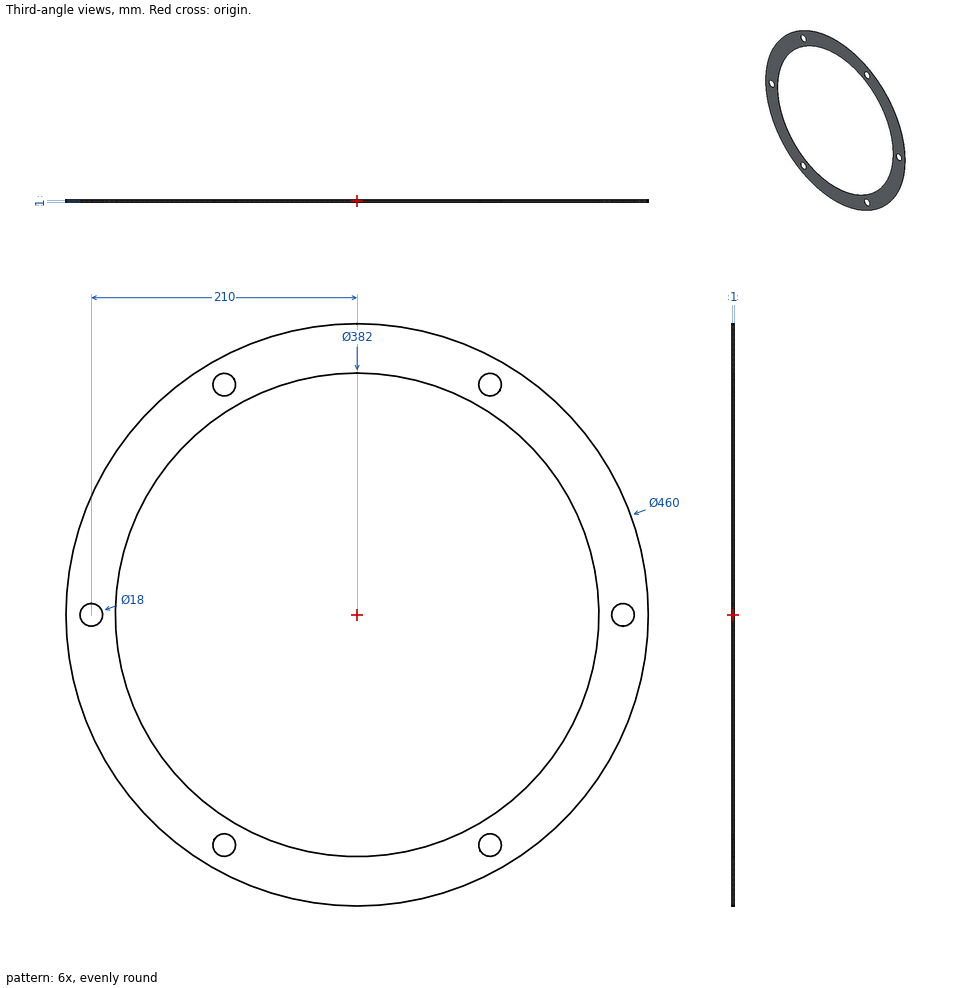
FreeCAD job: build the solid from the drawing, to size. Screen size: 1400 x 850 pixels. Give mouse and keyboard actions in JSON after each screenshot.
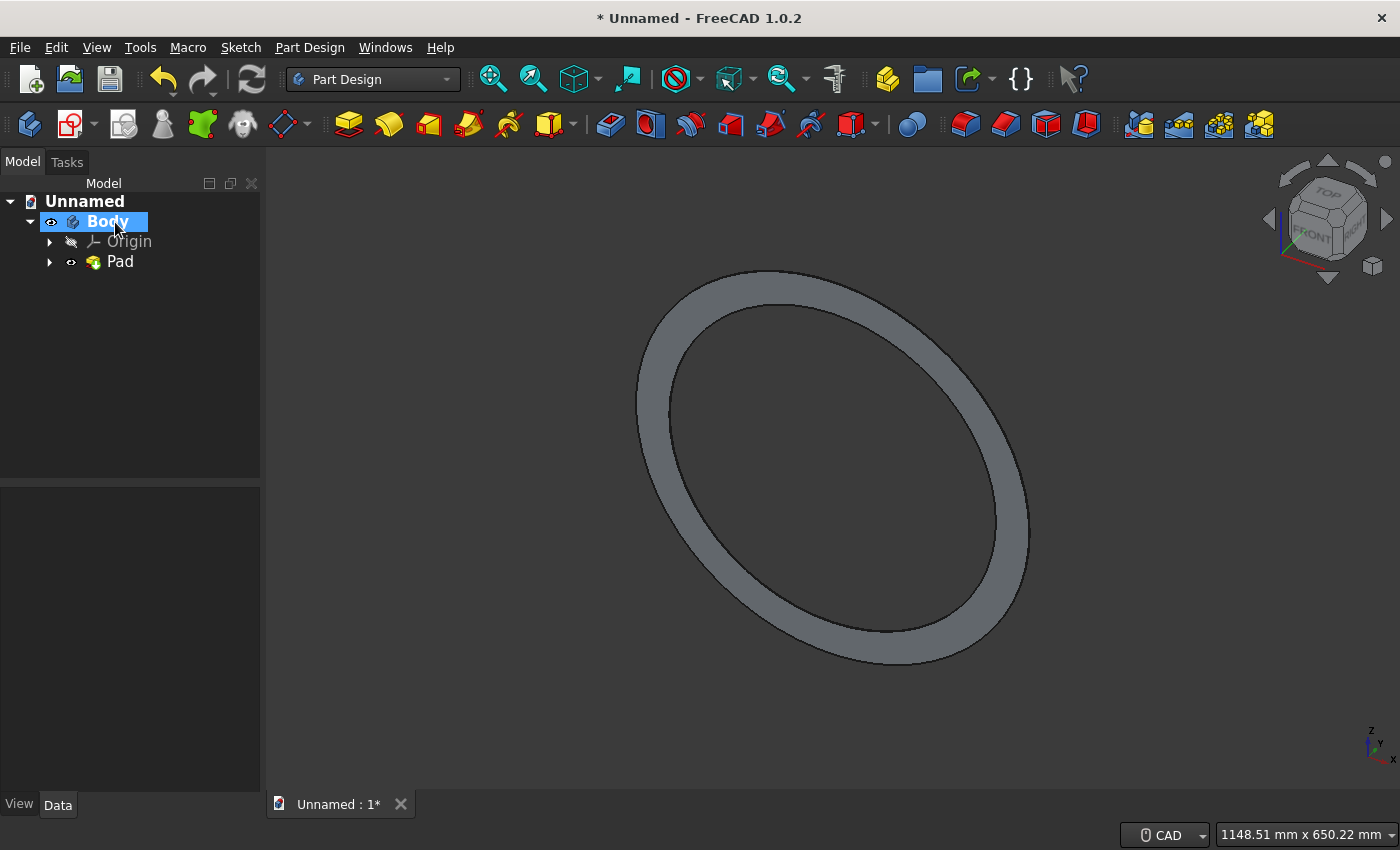
{"action": "left_click", "coordinate": [70, 124]}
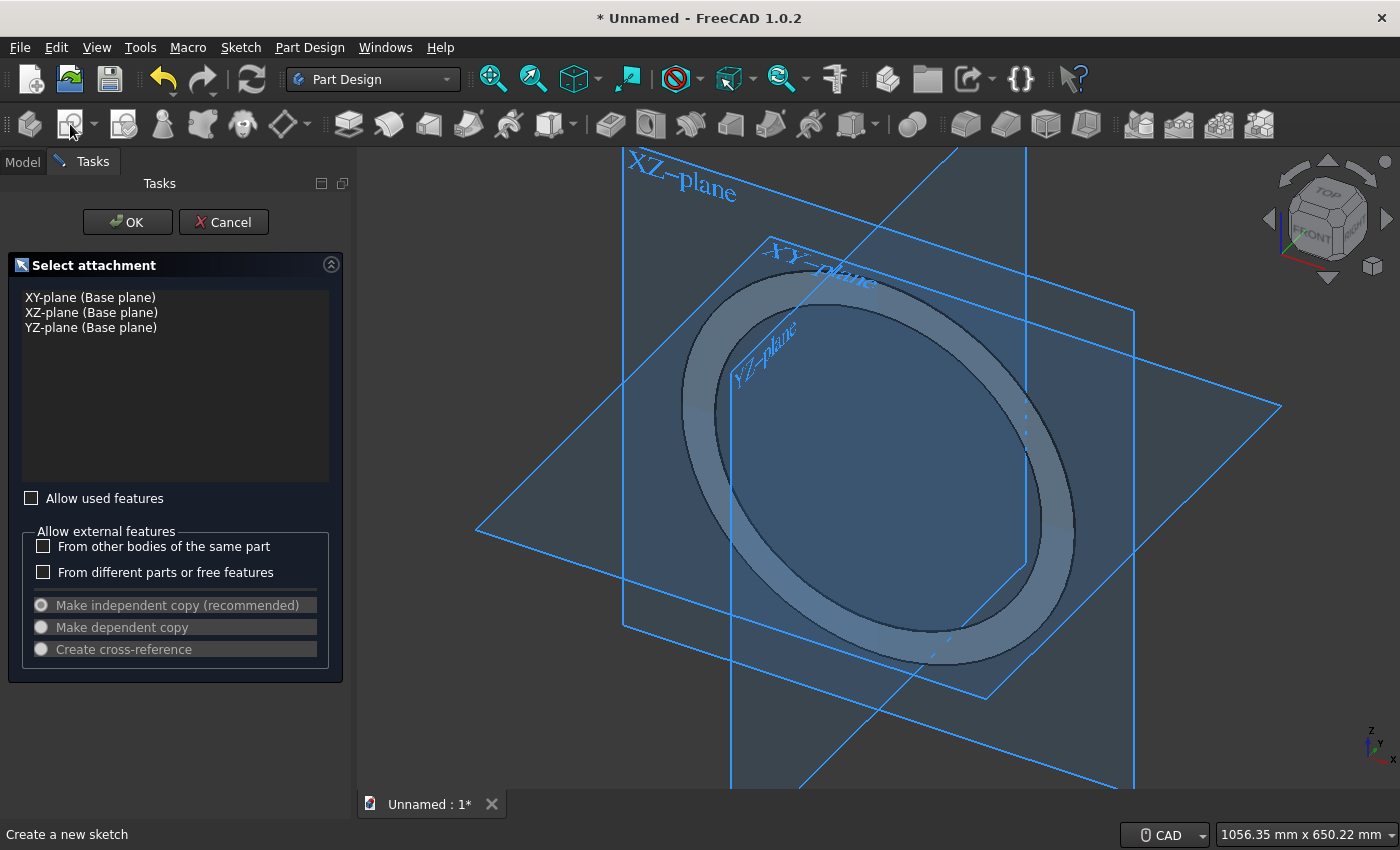
{"action": "left_click", "coordinate": [82, 312]}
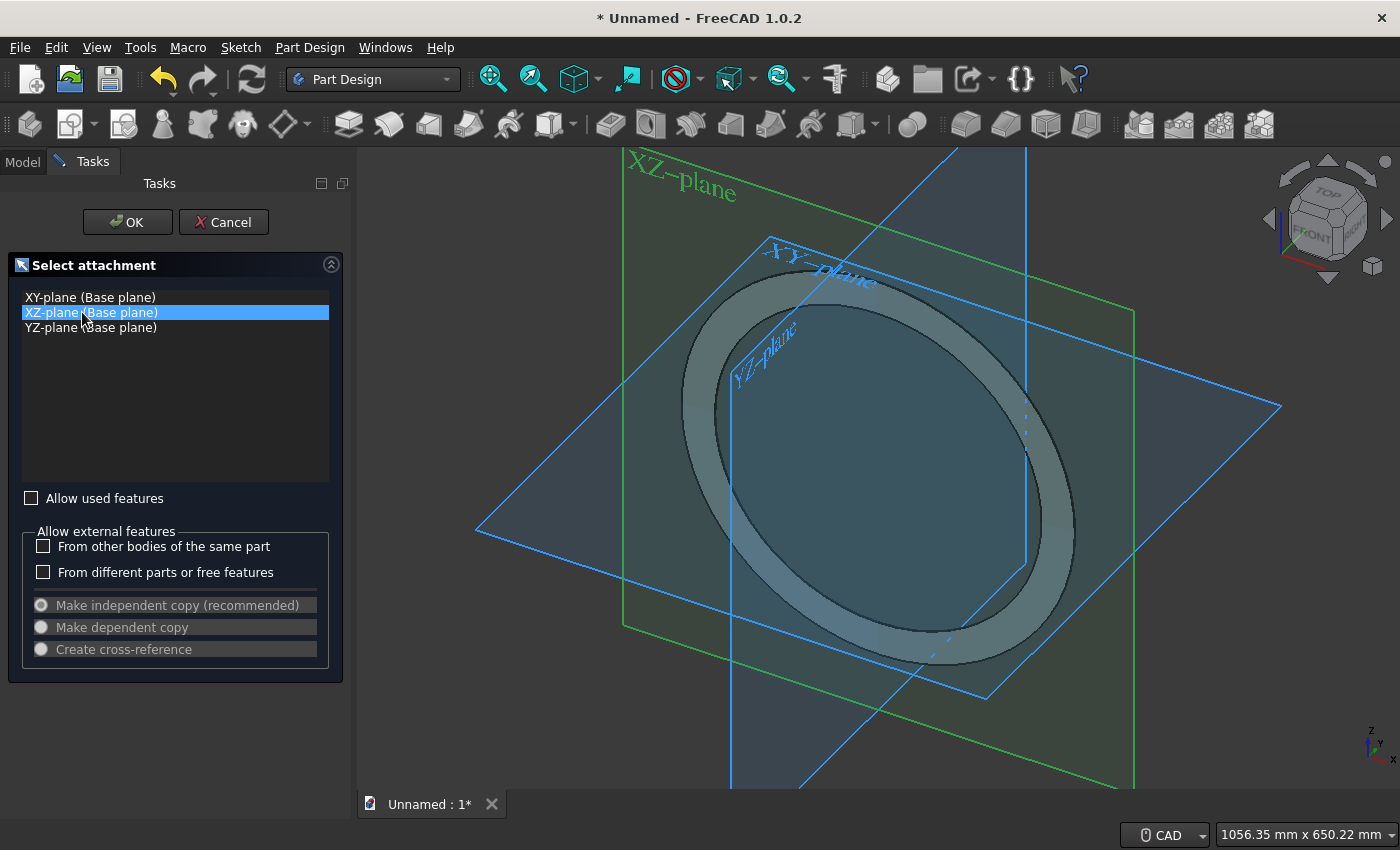
{"action": "left_click", "coordinate": [128, 222]}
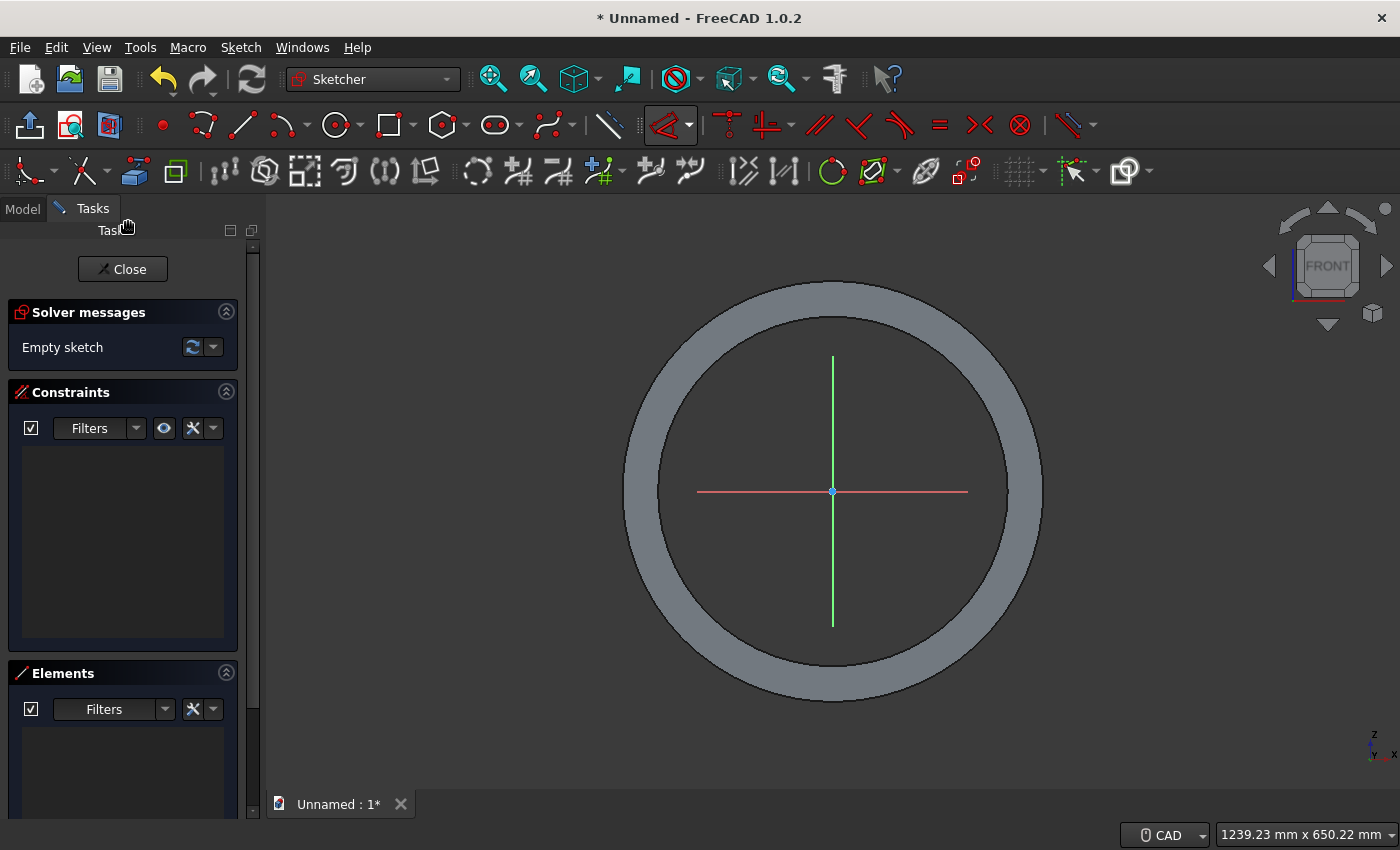
{"action": "key", "text": "q s"}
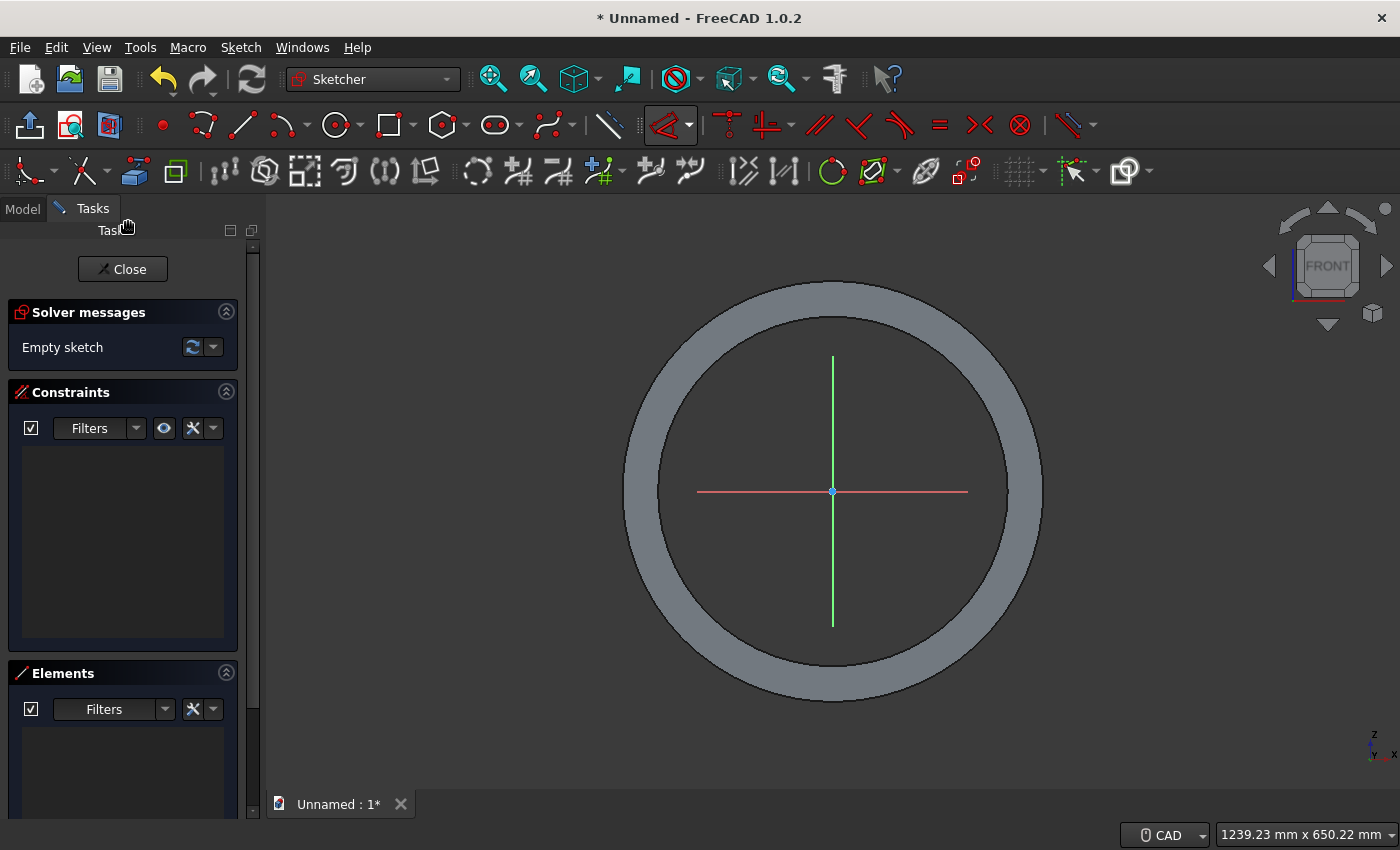
{"action": "scroll", "coordinate": [634, 492], "scroll_direction": "up", "scroll_amount": 15}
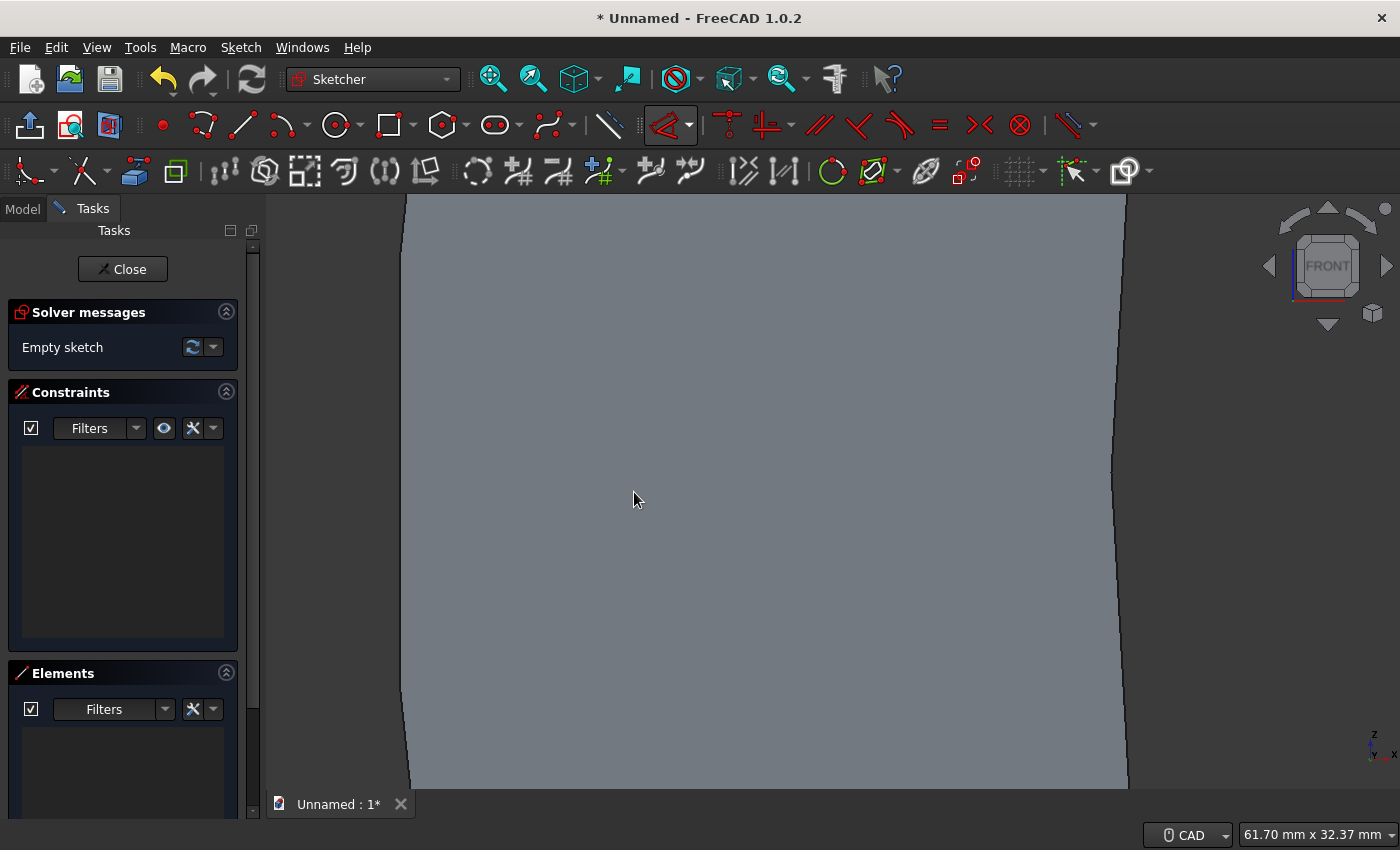
{"action": "key", "text": "g c"}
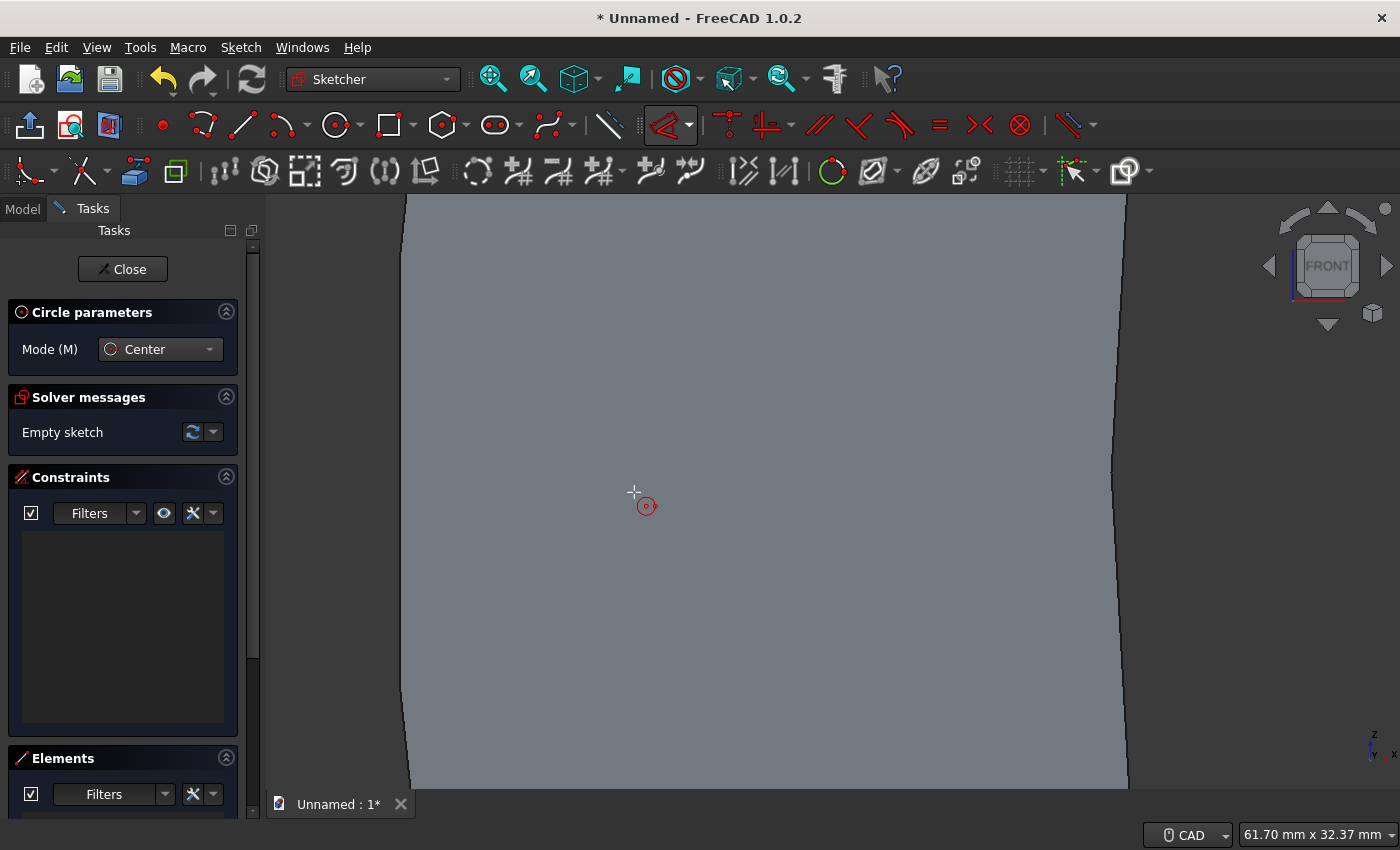
{"action": "left_click", "coordinate": [762, 472]}
{"action": "mouse_move", "coordinate": [879, 355]}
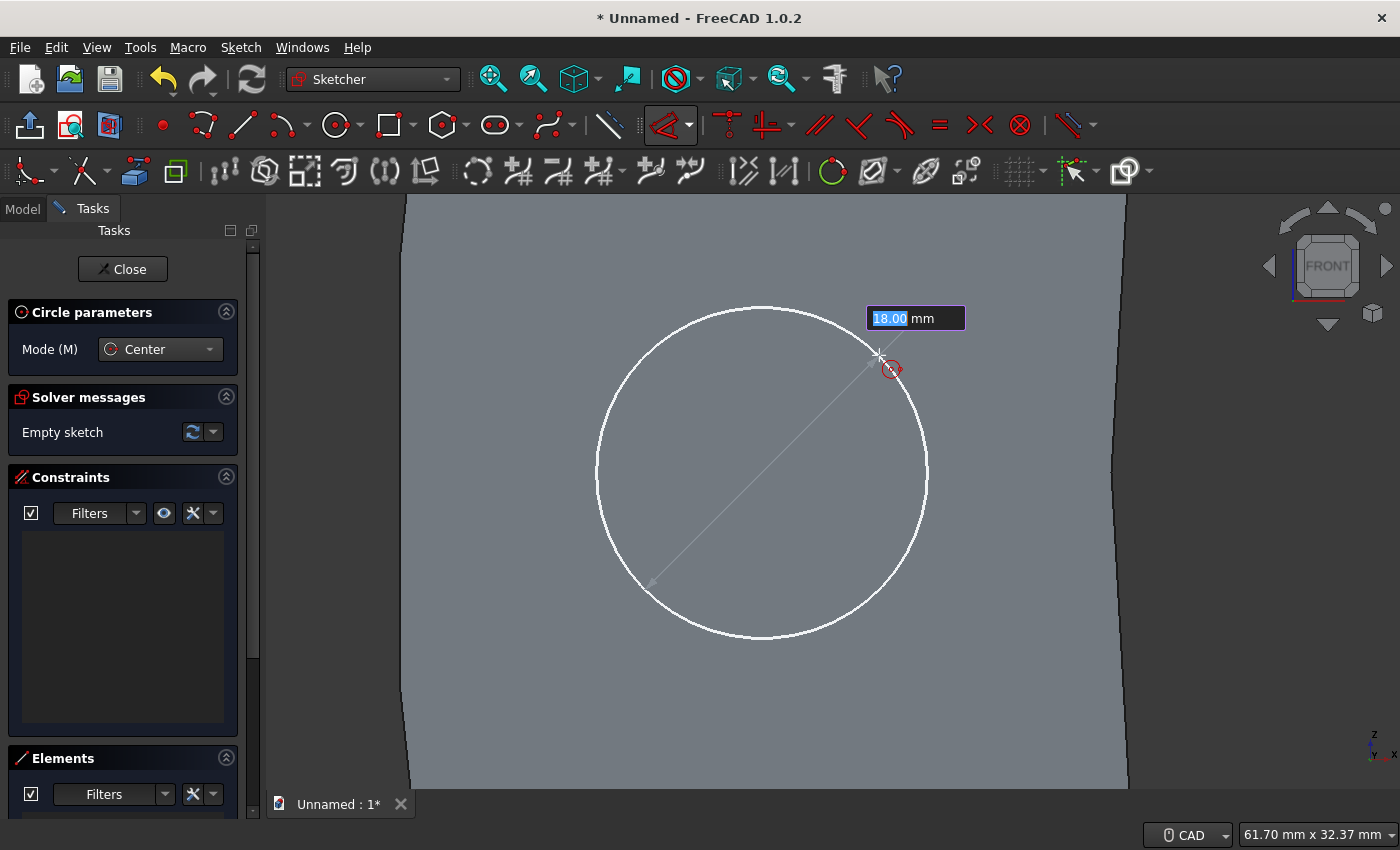
{"action": "type", "text": "18"}
{"action": "key", "text": "Return"}
{"action": "key", "text": "Escape"}